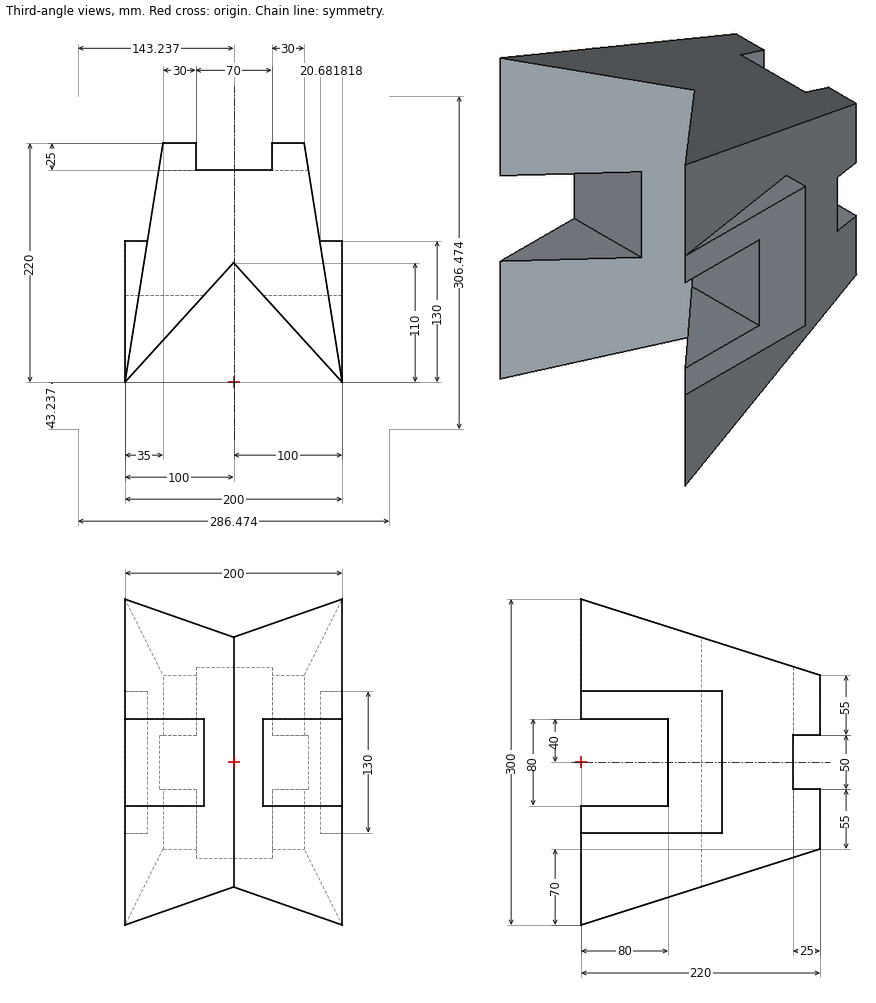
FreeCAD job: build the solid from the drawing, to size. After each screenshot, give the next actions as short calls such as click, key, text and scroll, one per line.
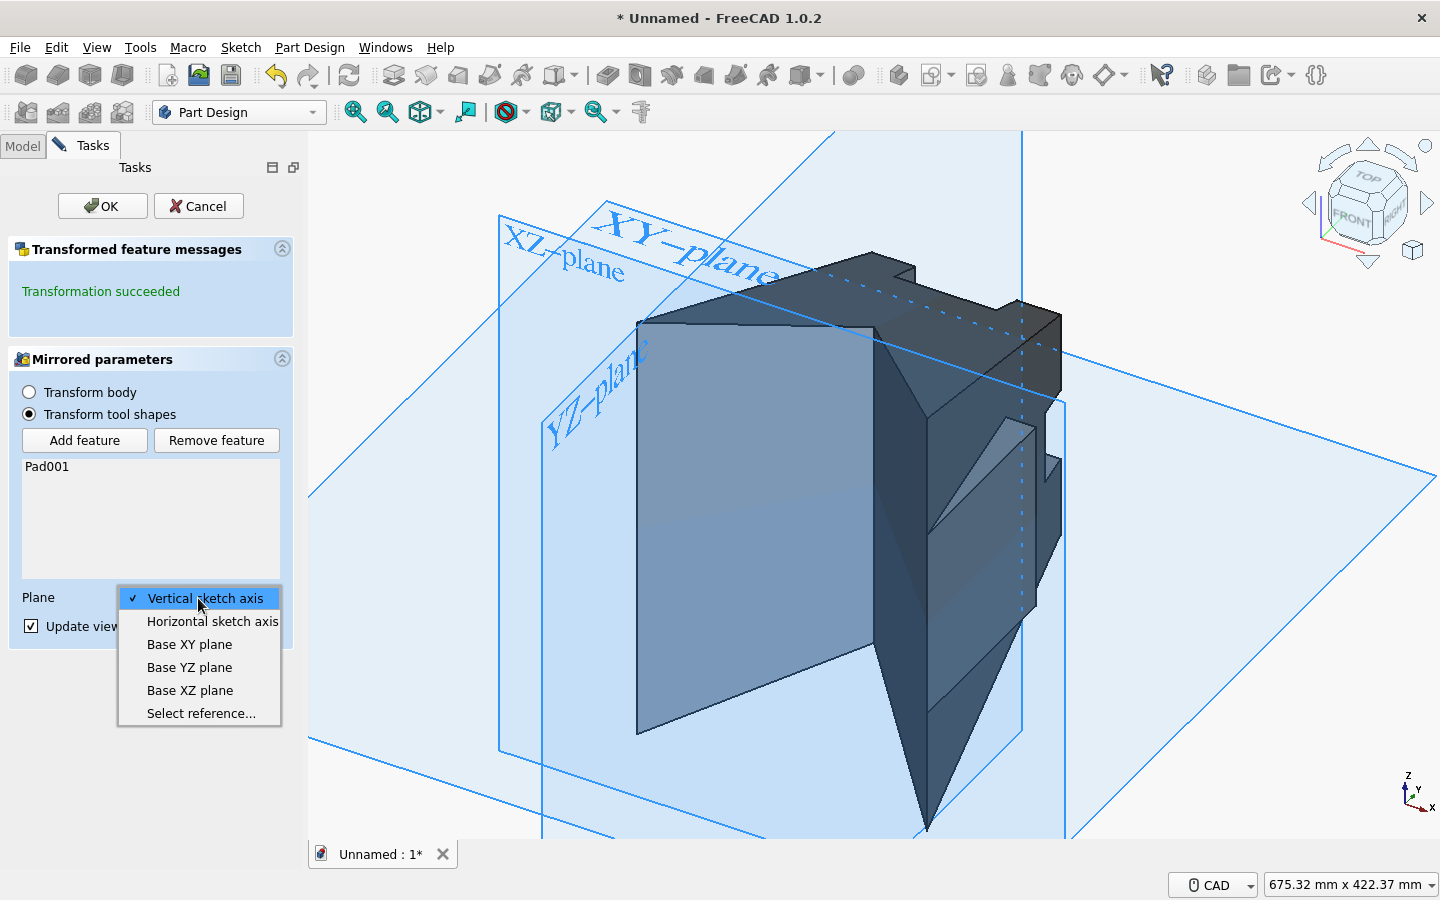
click(198, 668)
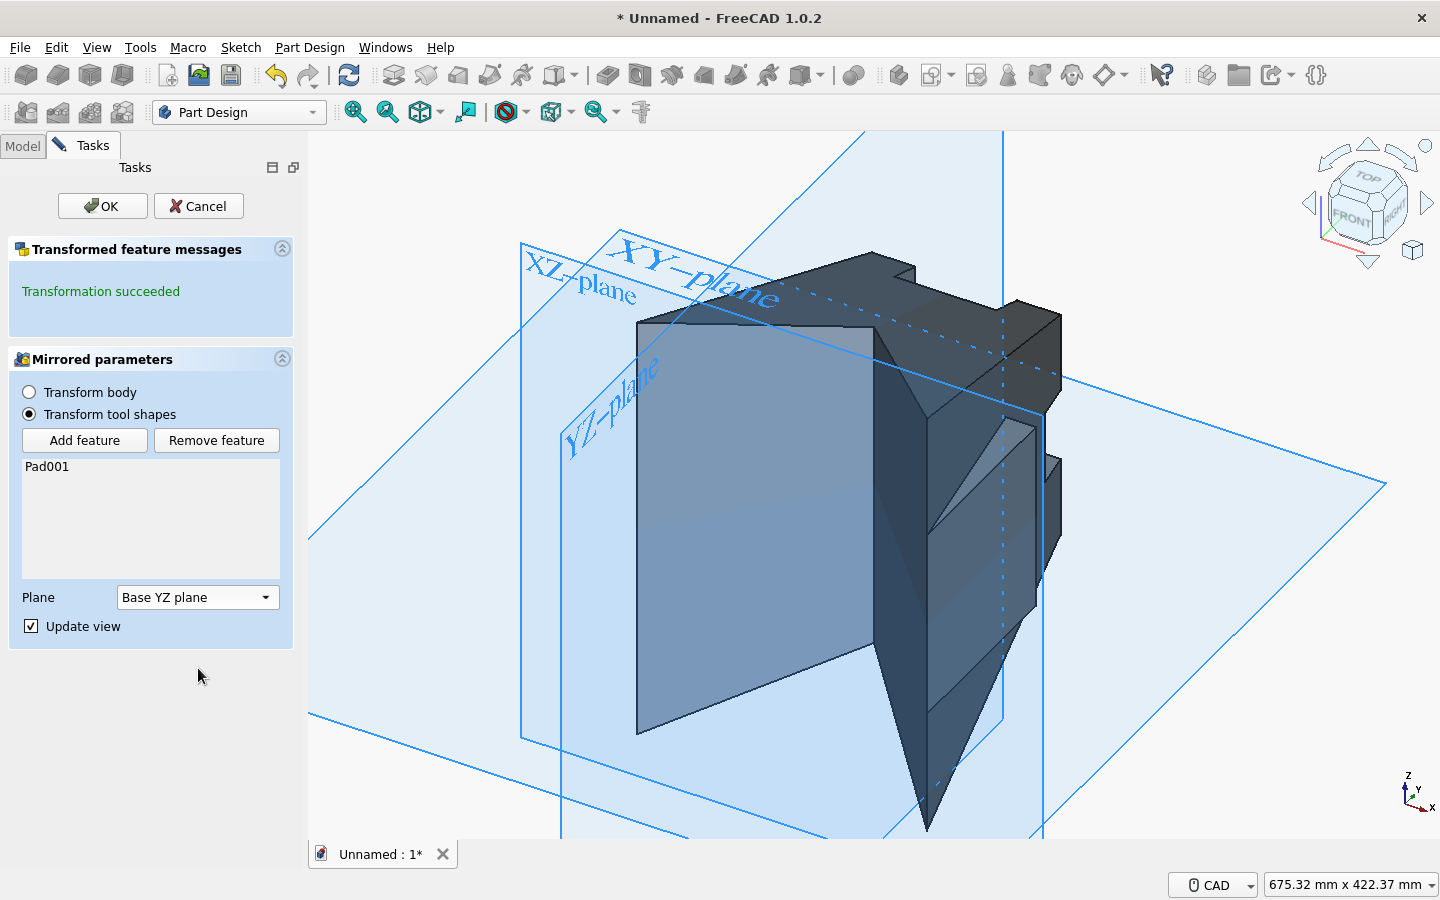
click(103, 206)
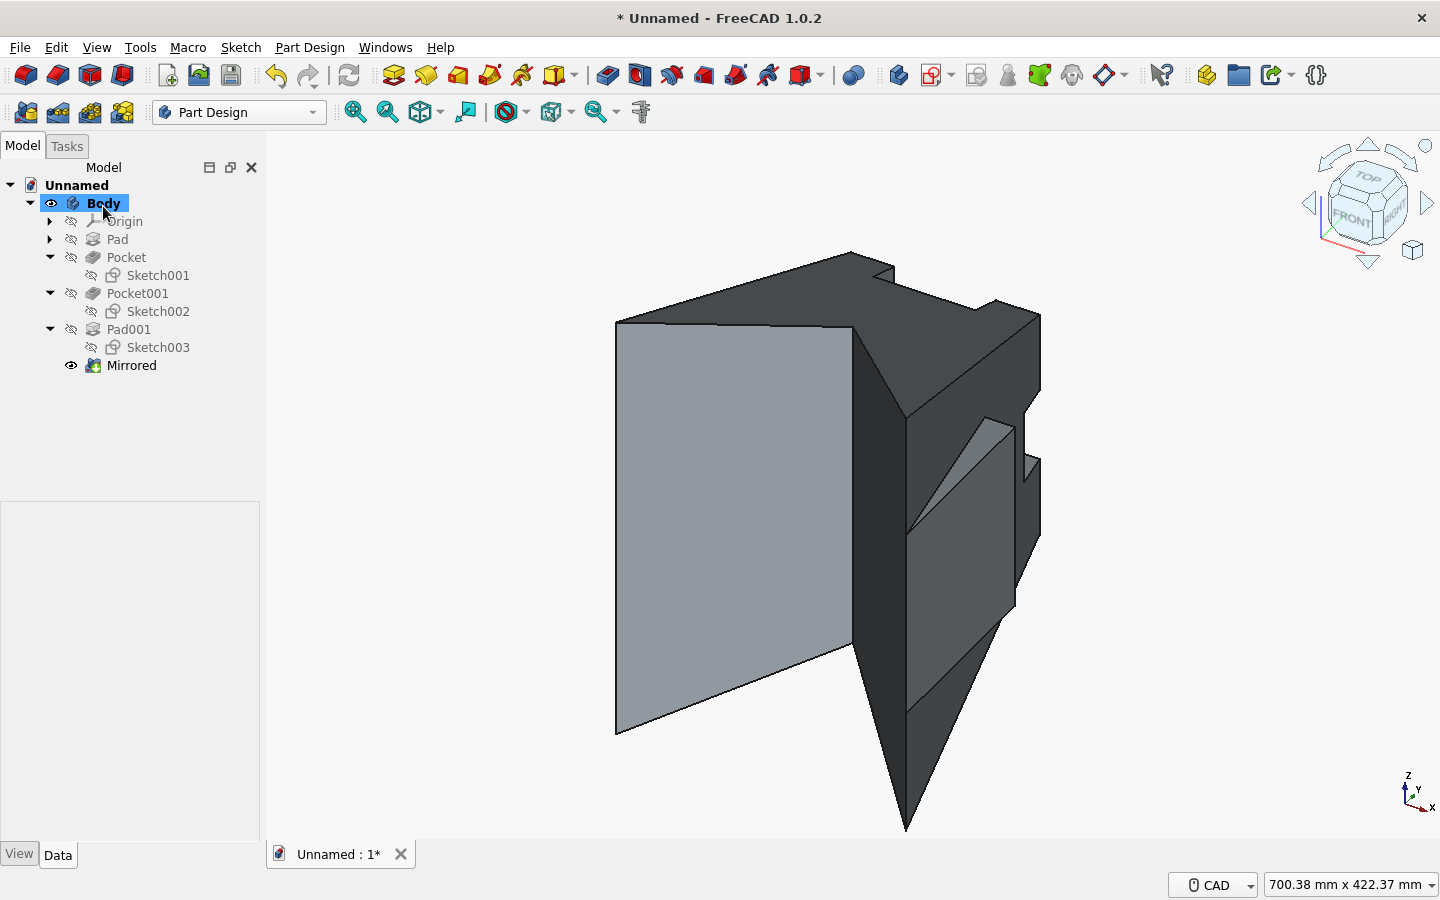
click(960, 570)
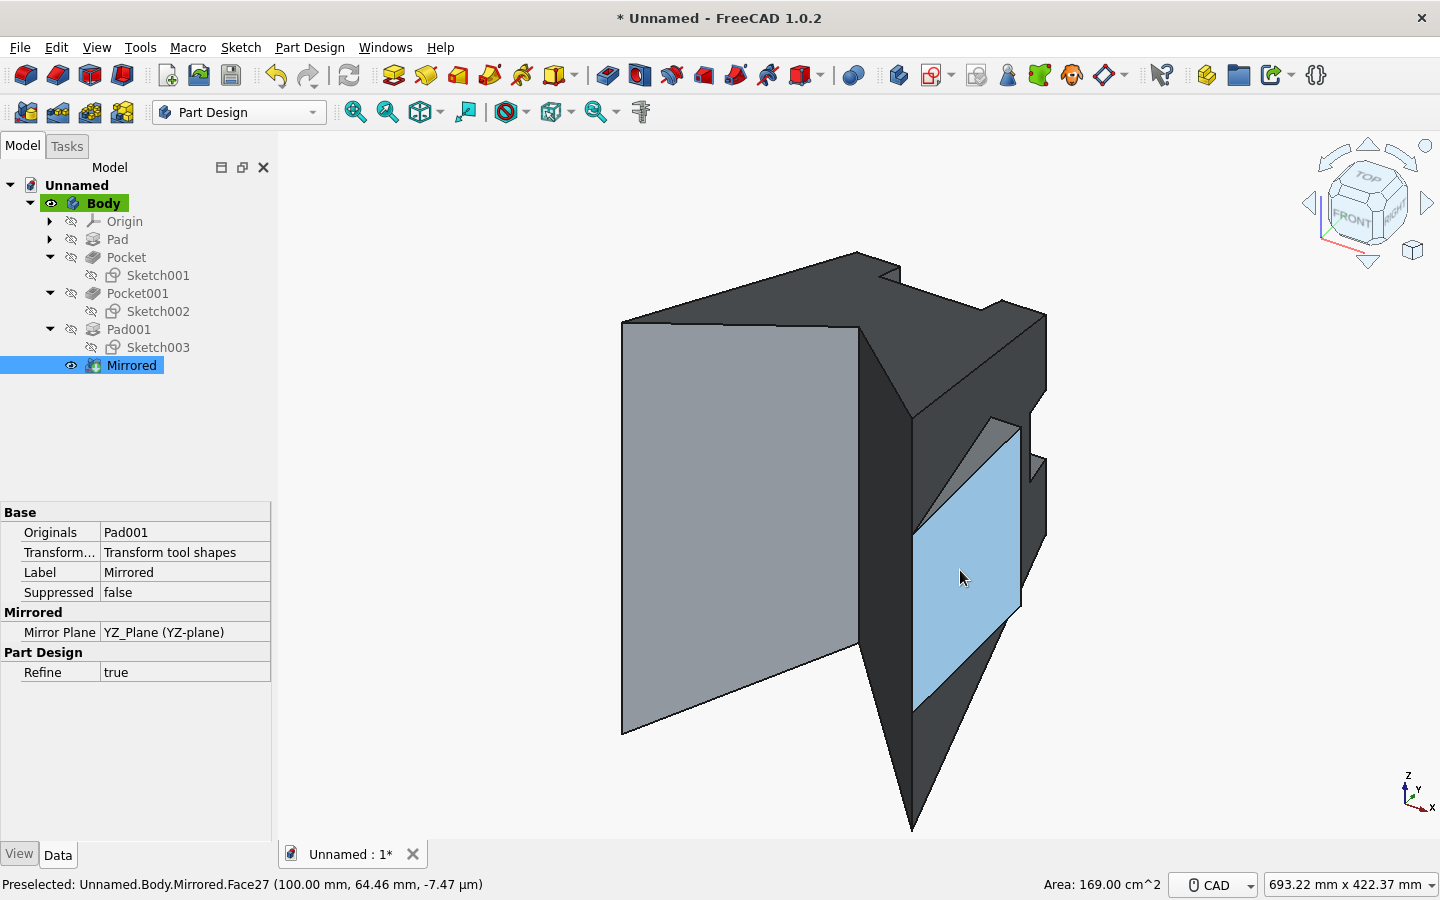
click(932, 76)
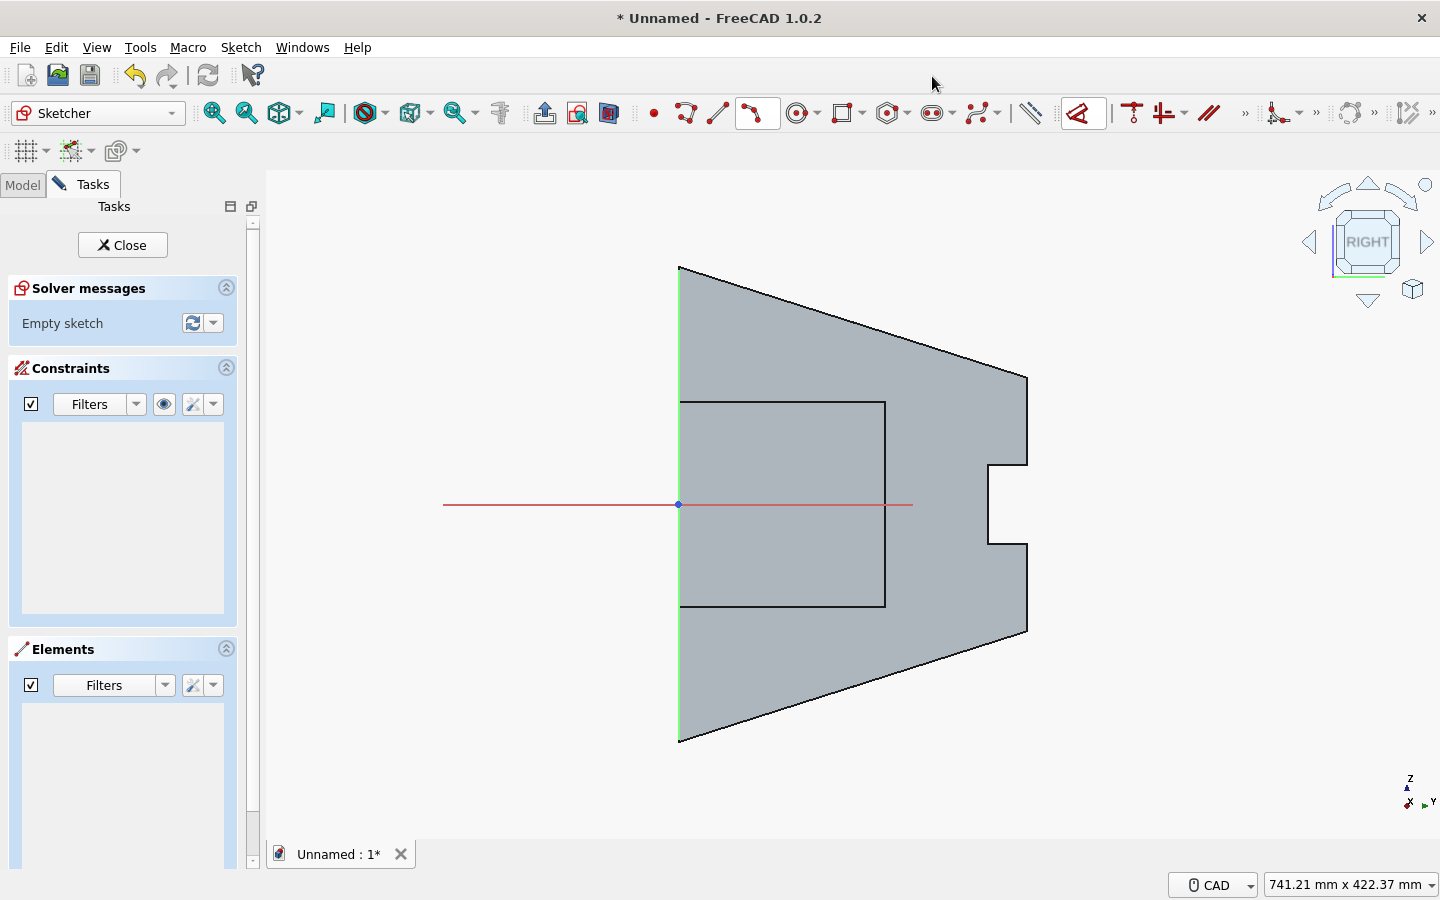
scroll(724, 504, up, 6)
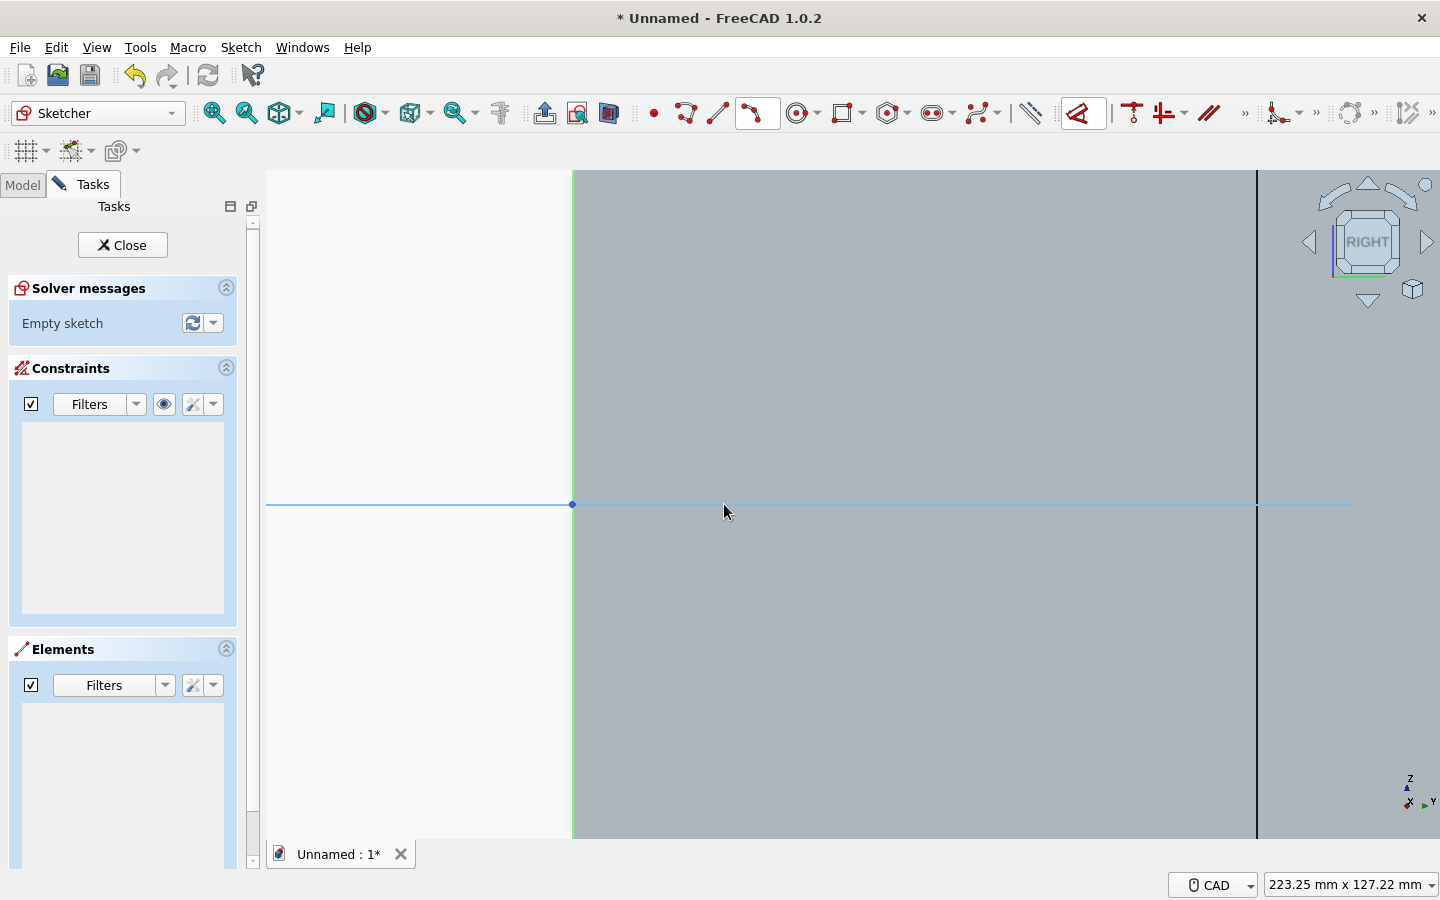
key(g)
key(r)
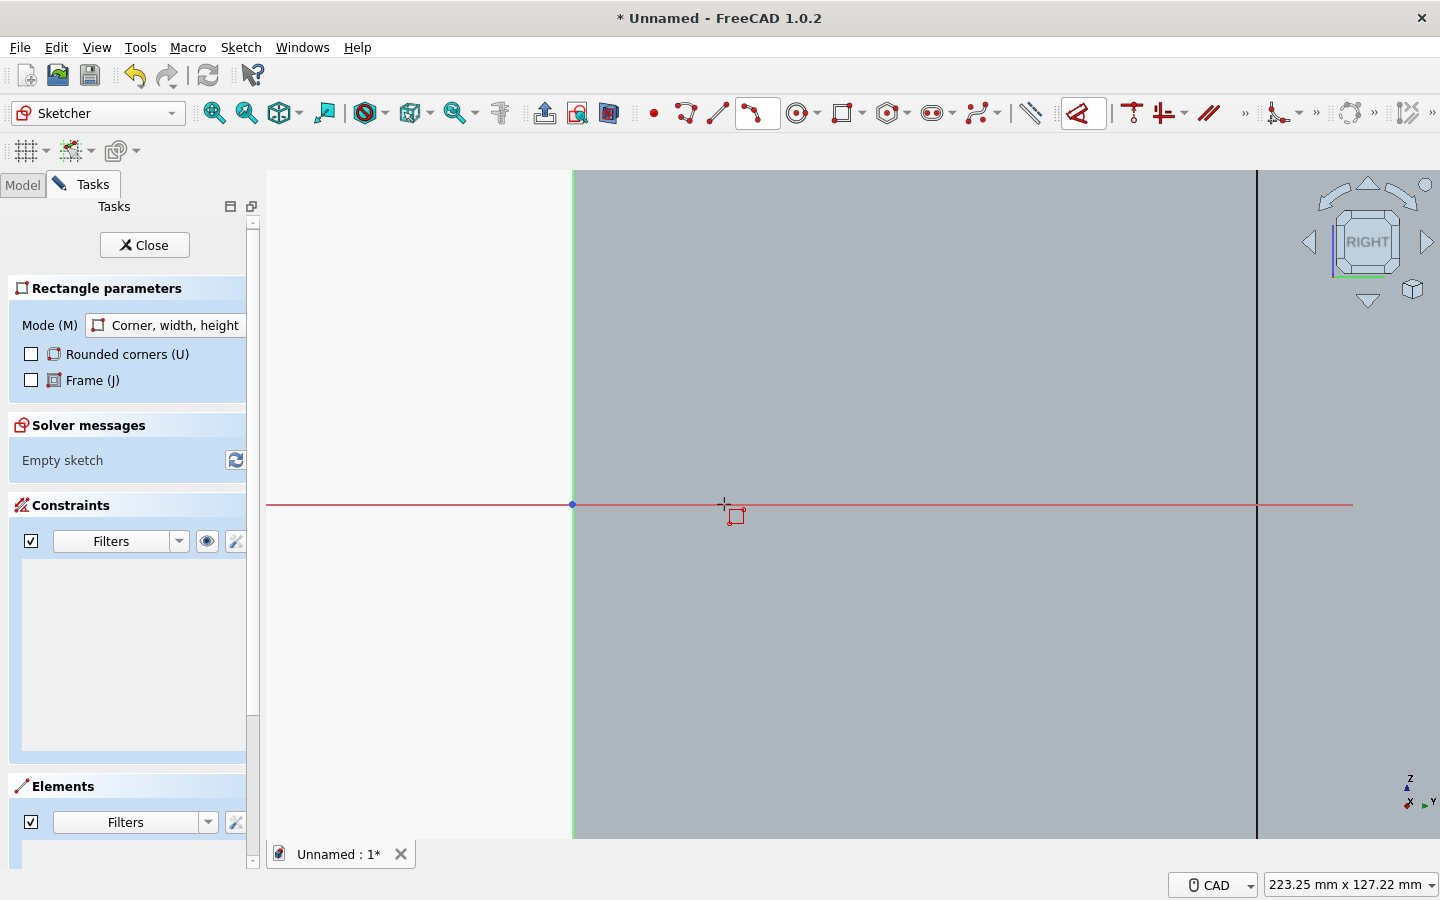
click(573, 294)
move(994, 715)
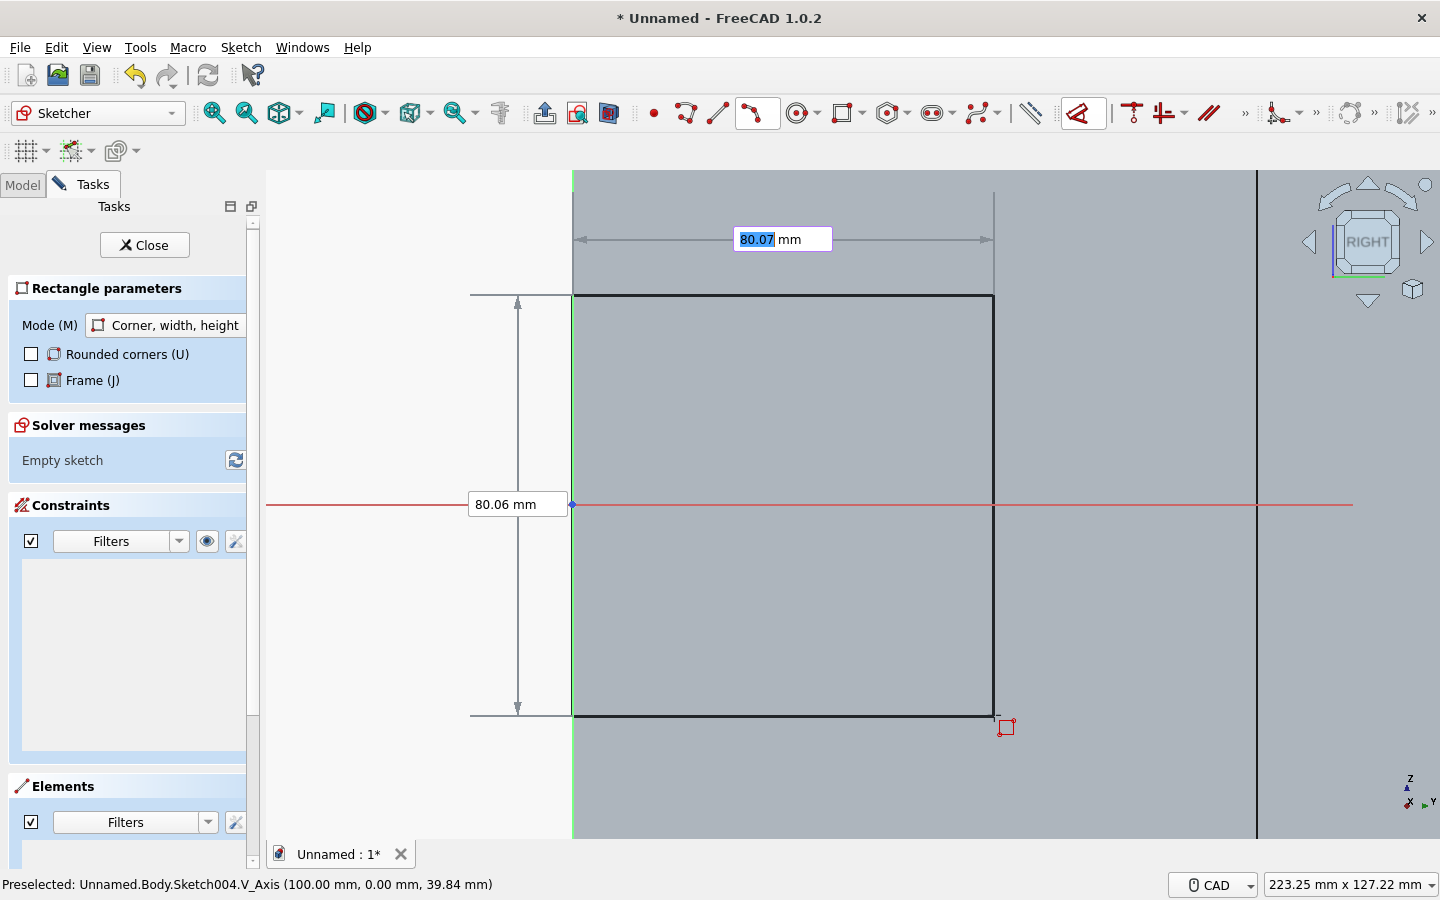
text(80)
key(Tab)
text(80)
key(Return)
key(Escape)